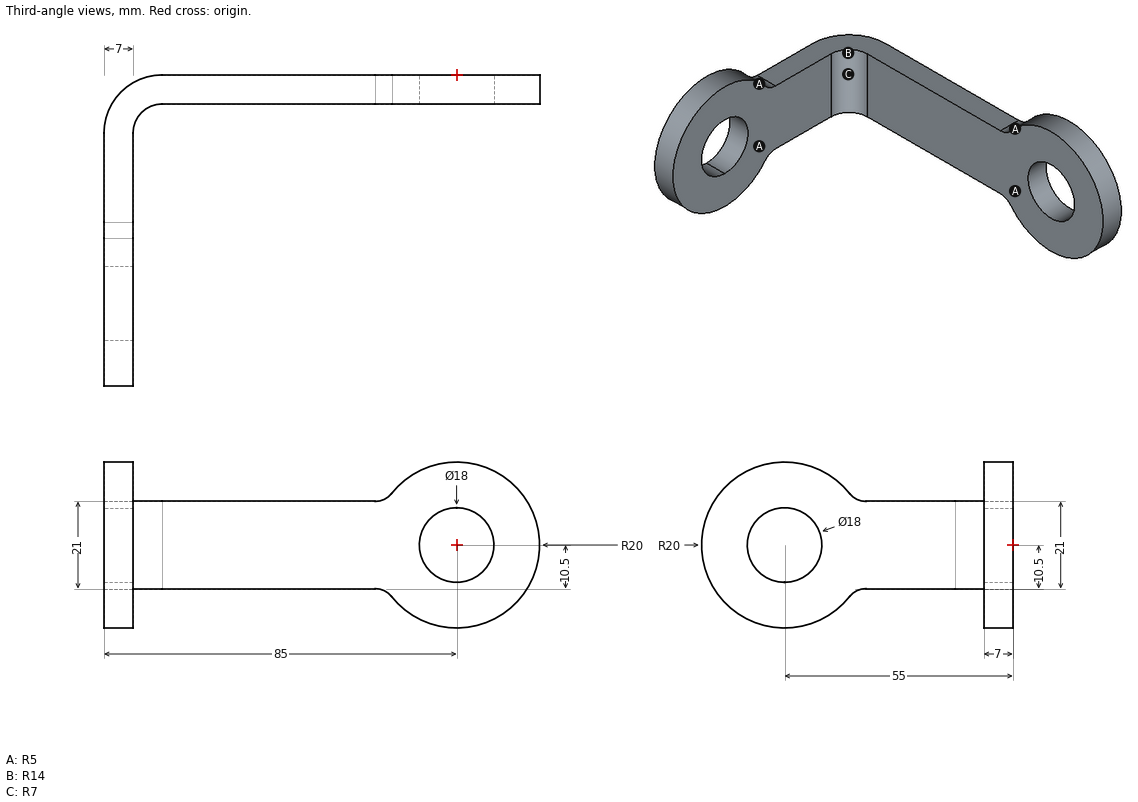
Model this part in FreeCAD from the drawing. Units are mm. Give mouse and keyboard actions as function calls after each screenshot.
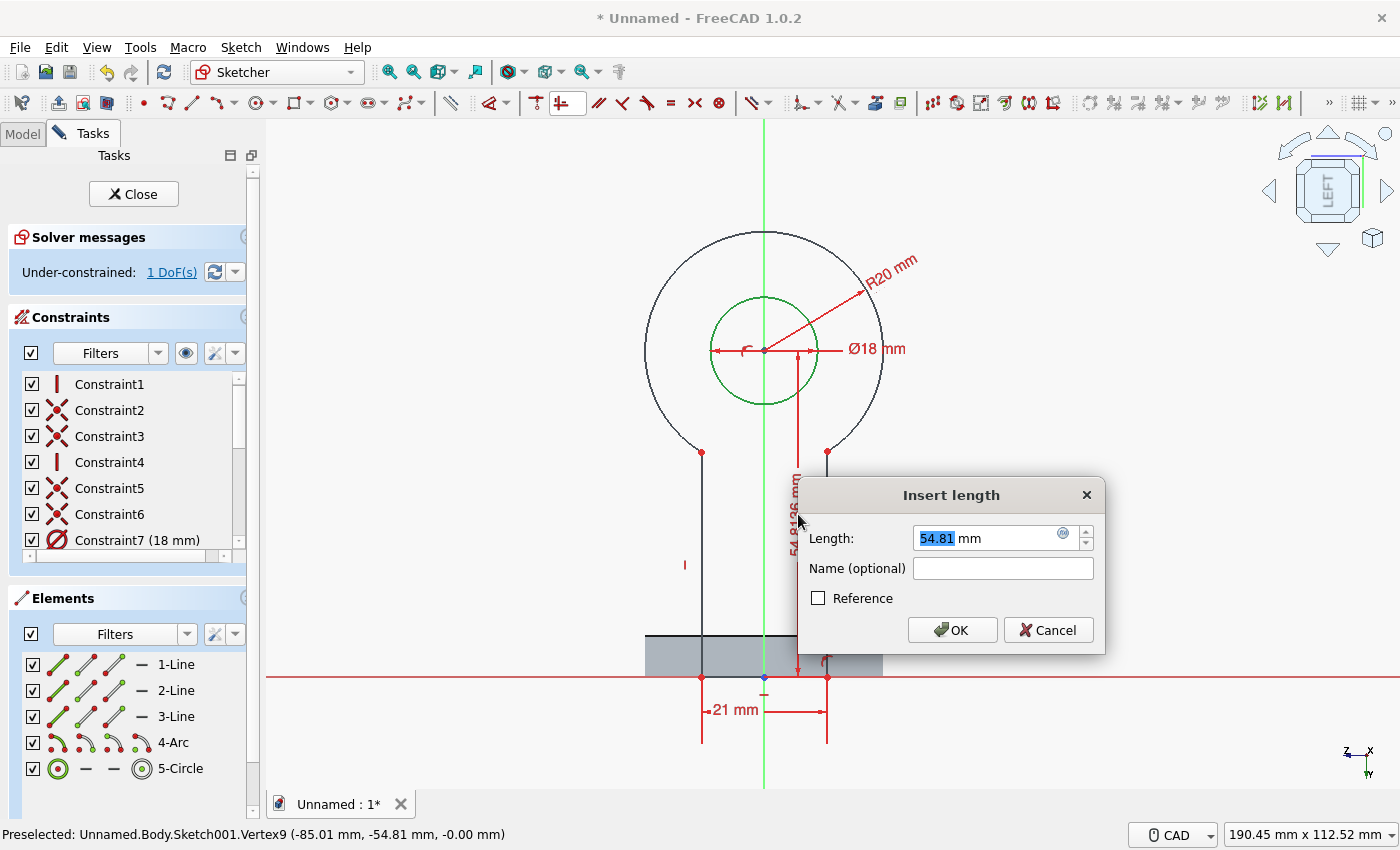
text(55)
key(Return)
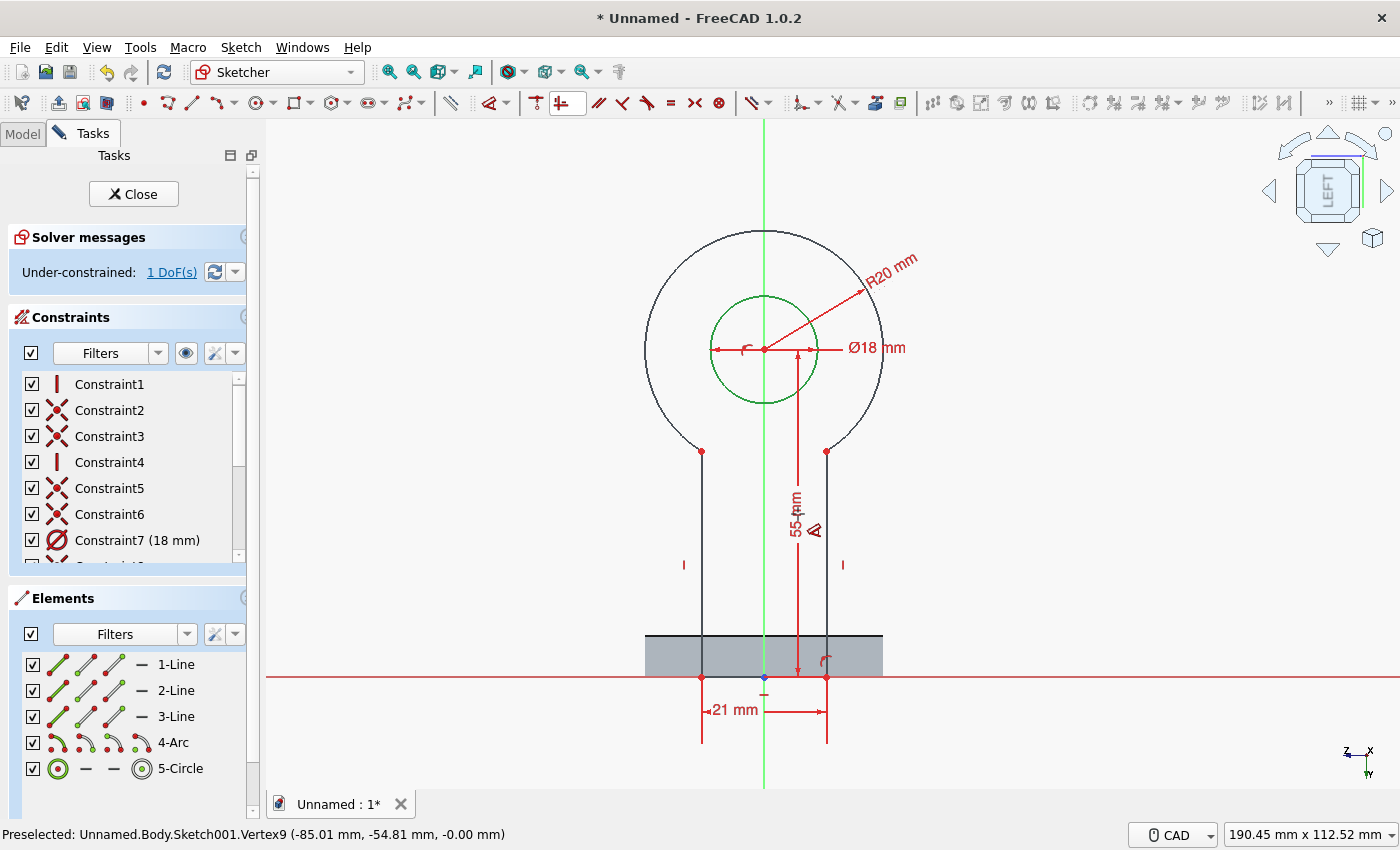
click(827, 451)
click(810, 711)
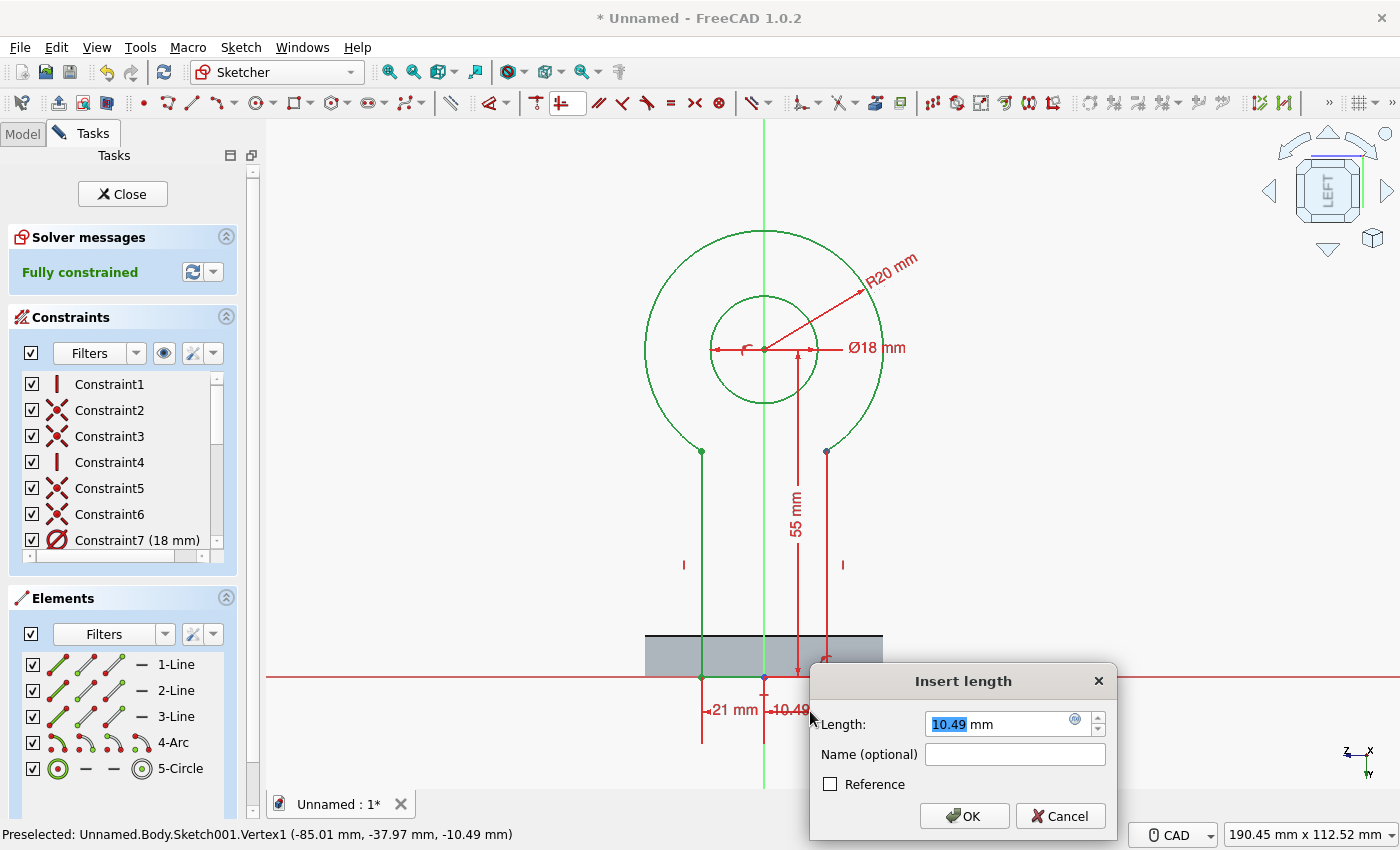
text(10.5)
key(Return)
key(Escape)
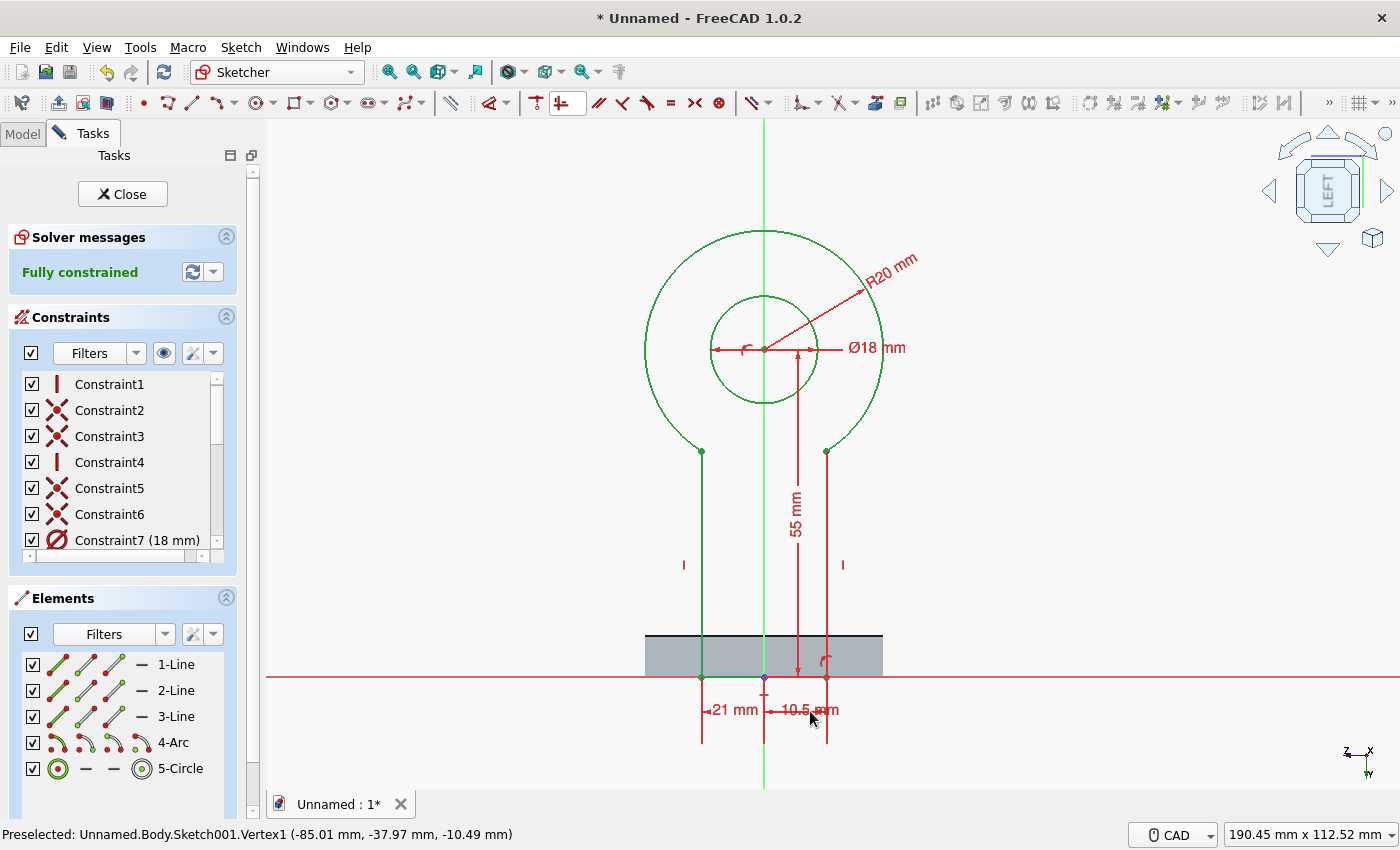
click(123, 194)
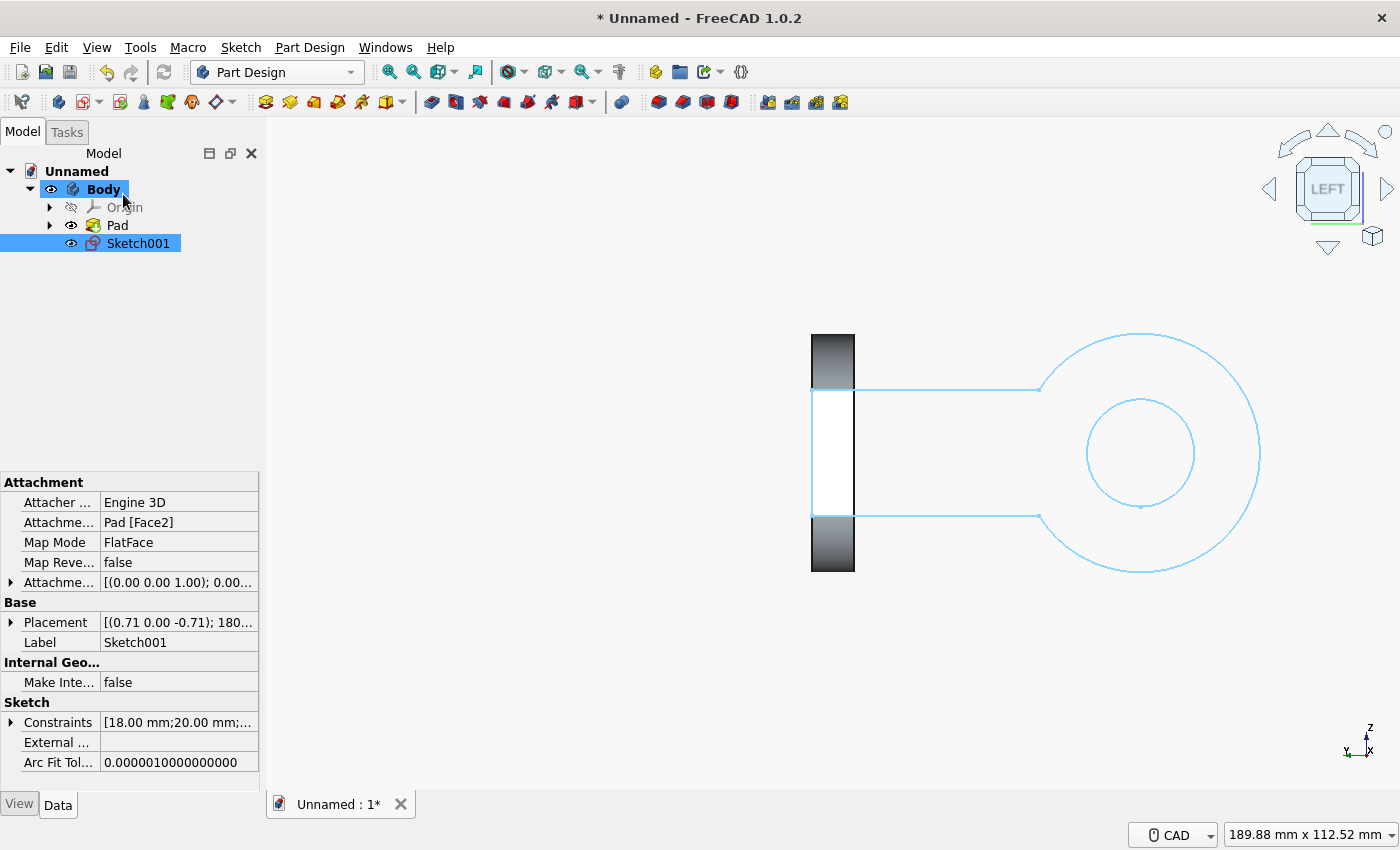
click(266, 102)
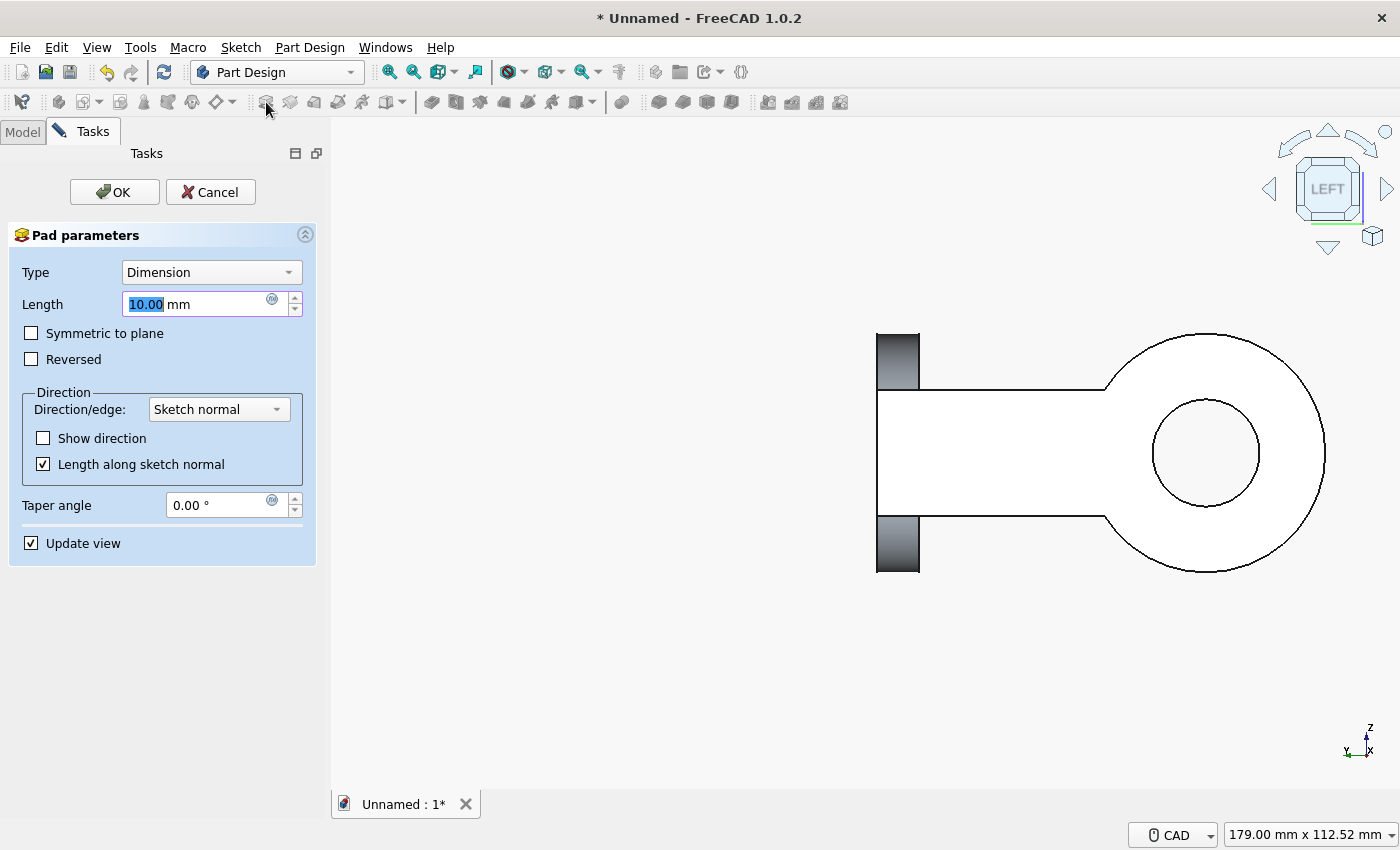
text(7)
key(Tab)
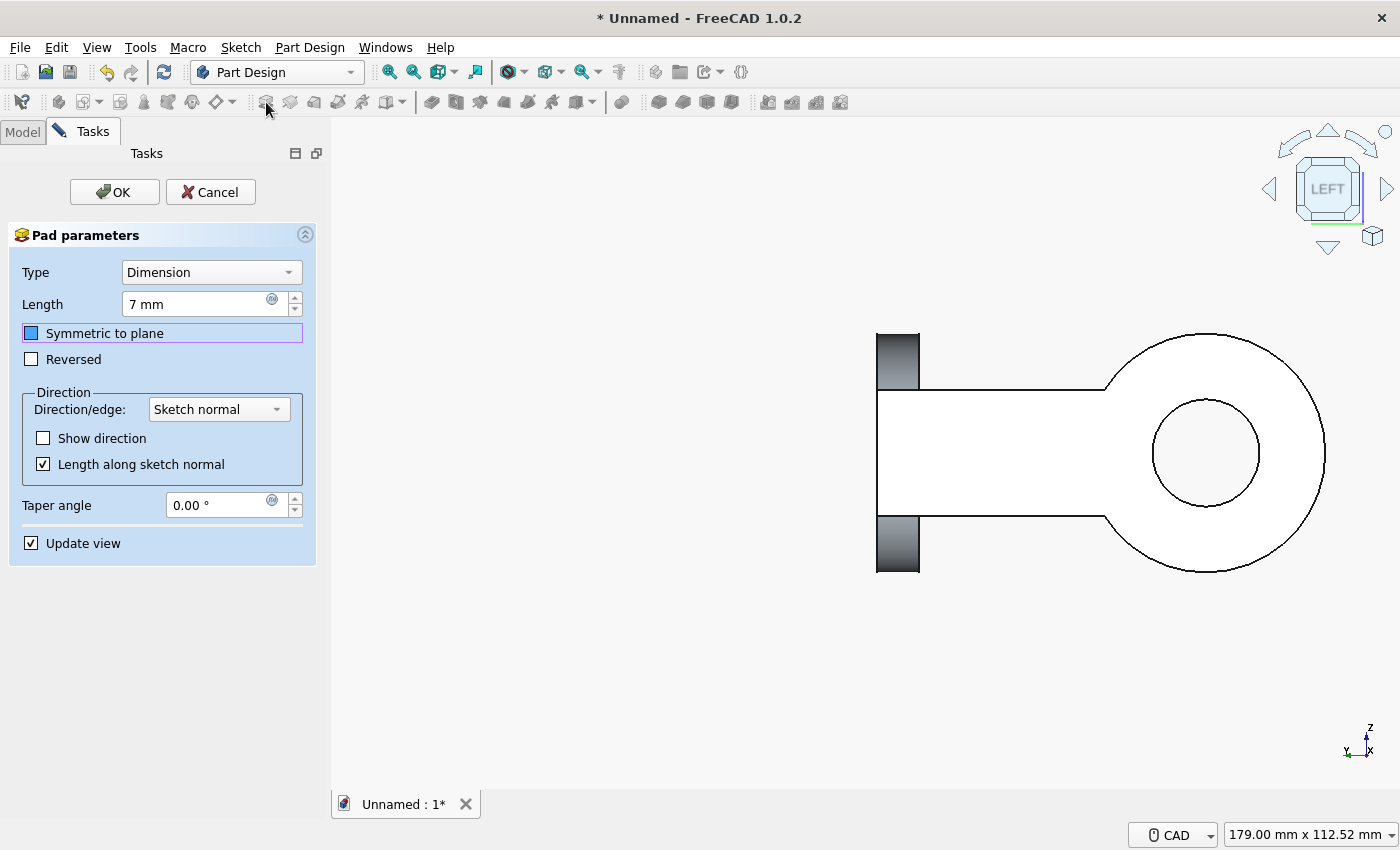
click(30, 359)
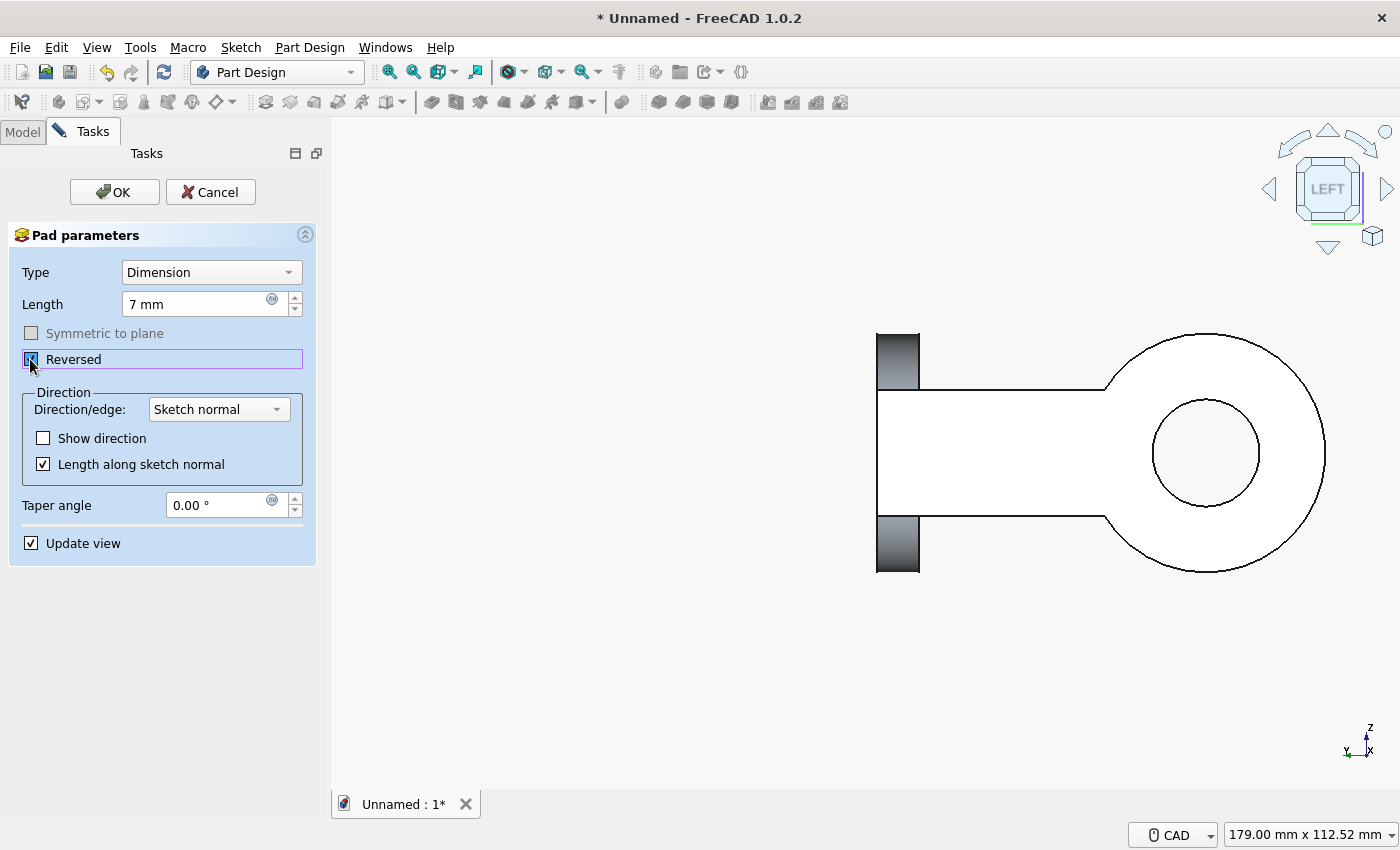
click(115, 192)